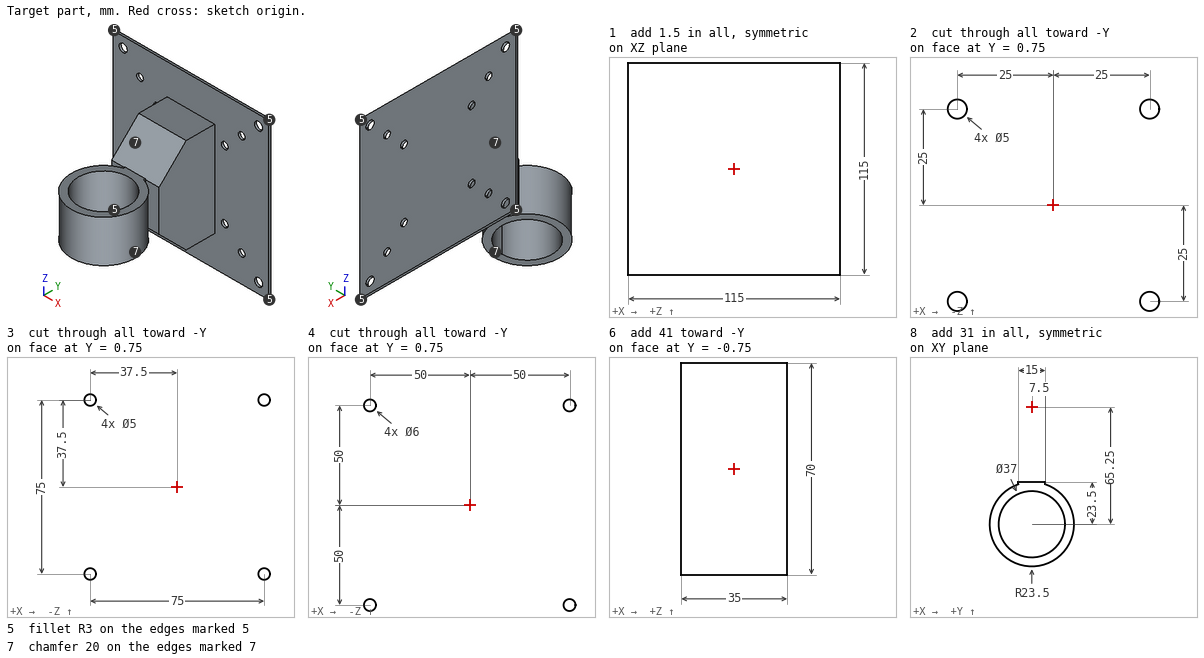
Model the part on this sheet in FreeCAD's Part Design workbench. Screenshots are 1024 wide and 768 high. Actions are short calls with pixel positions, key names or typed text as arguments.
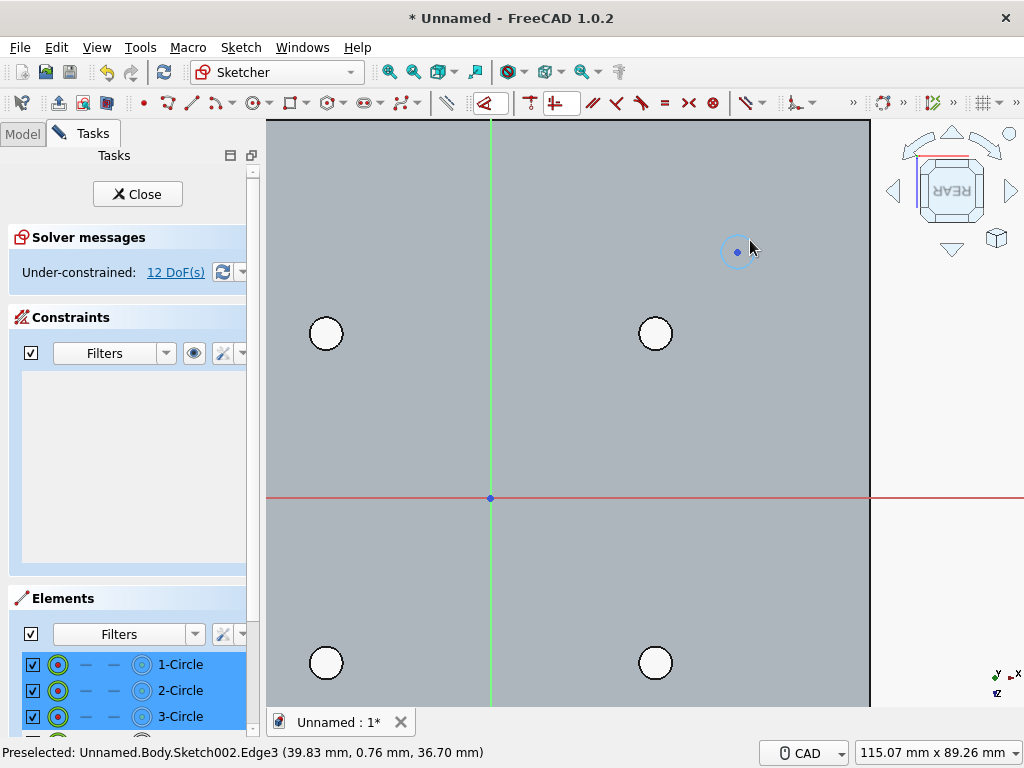
click(749, 240)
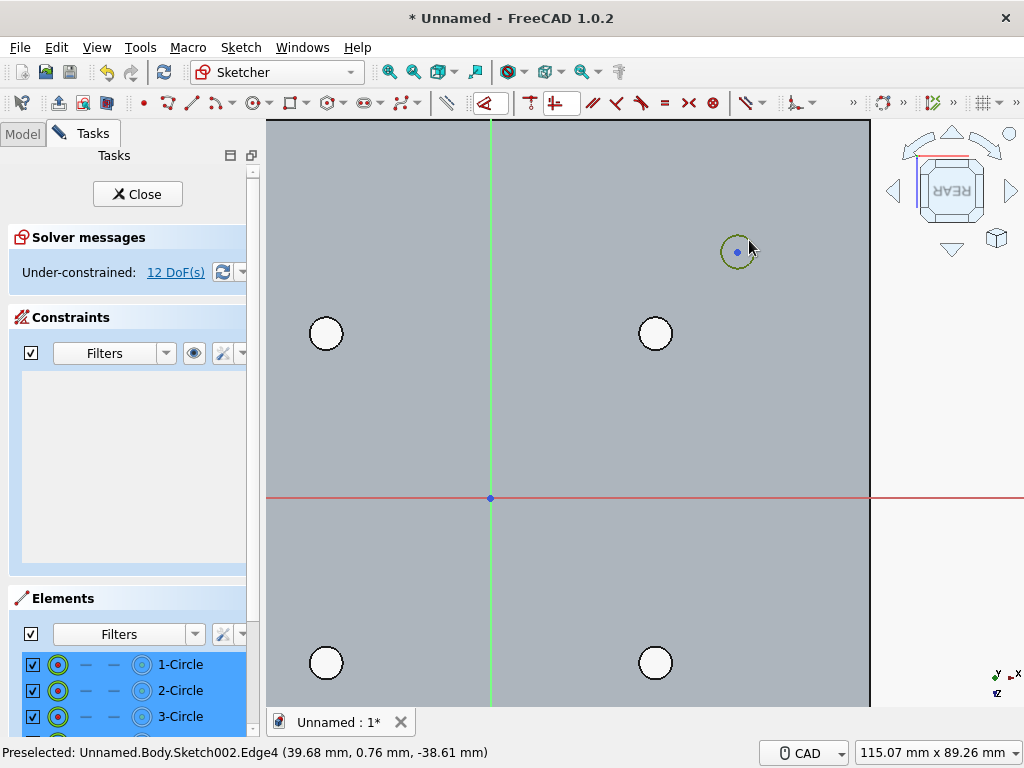
key(e)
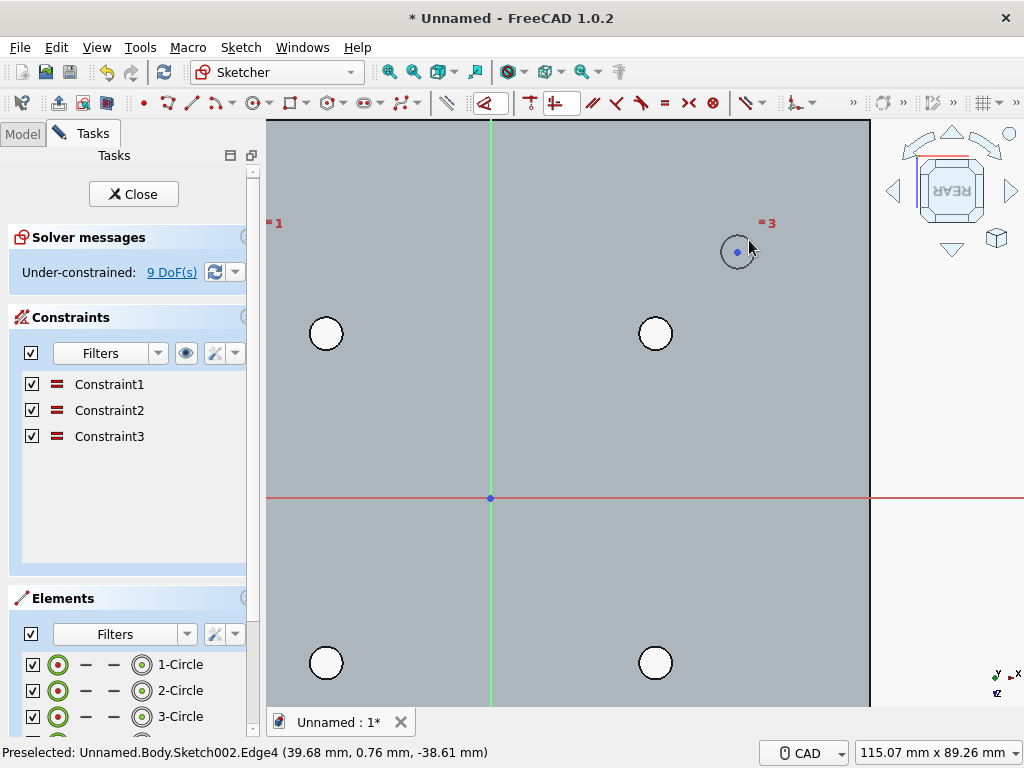
scroll(750, 239, down, 2)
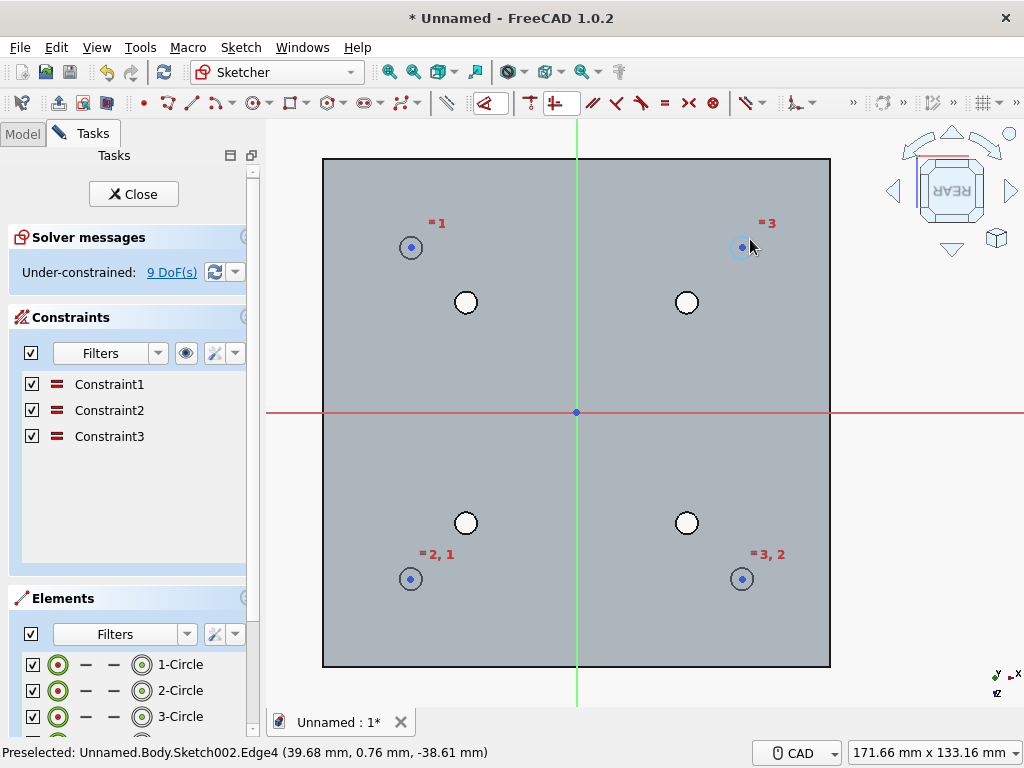
click(411, 248)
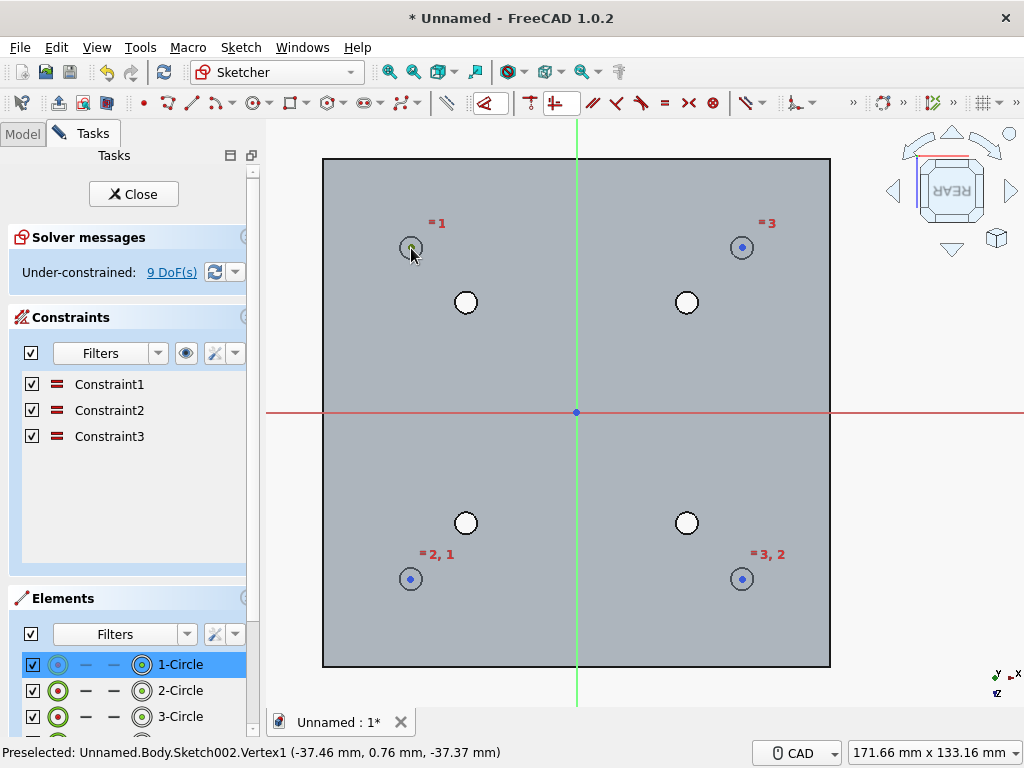
click(411, 579)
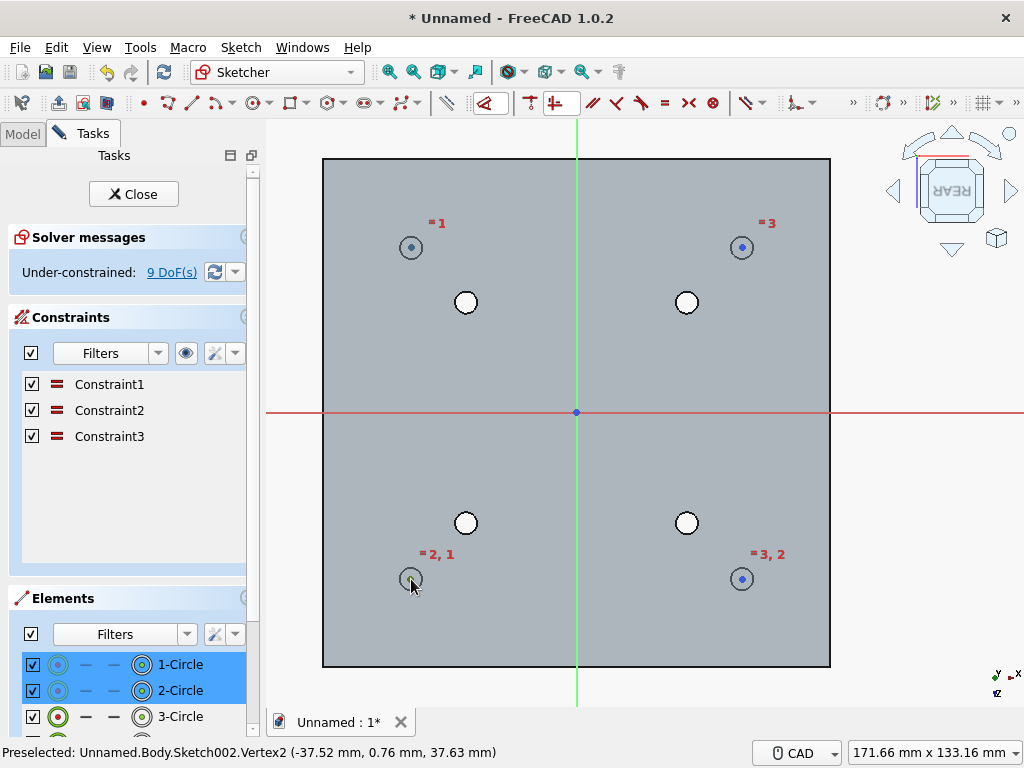
key(v)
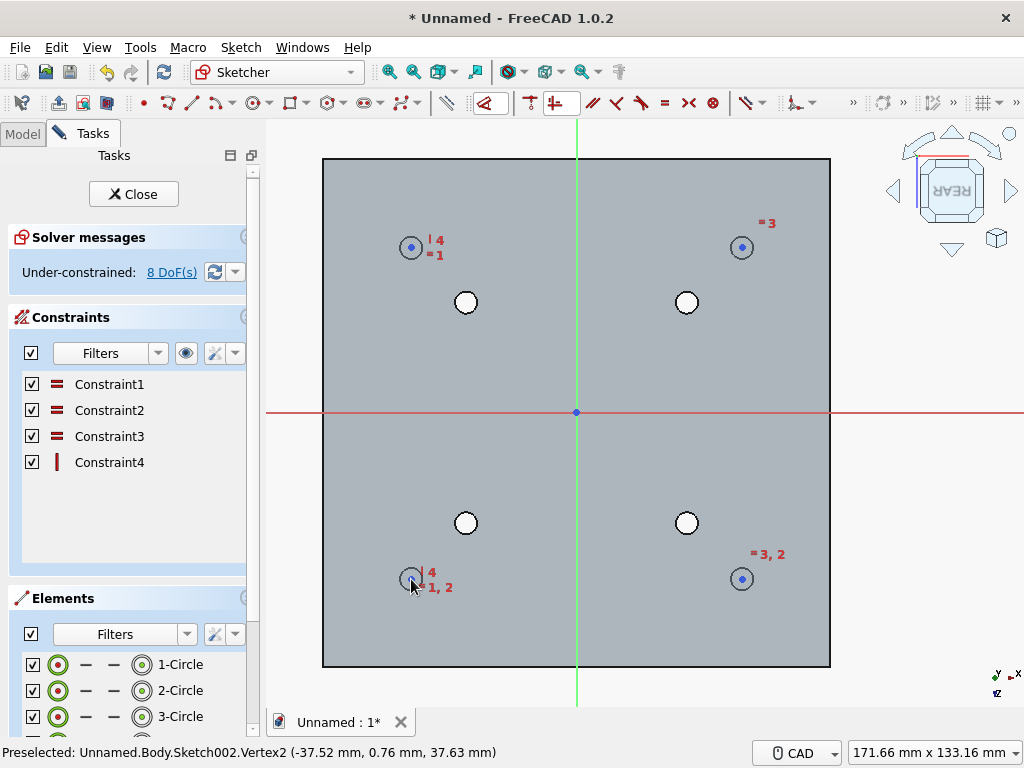
click(411, 579)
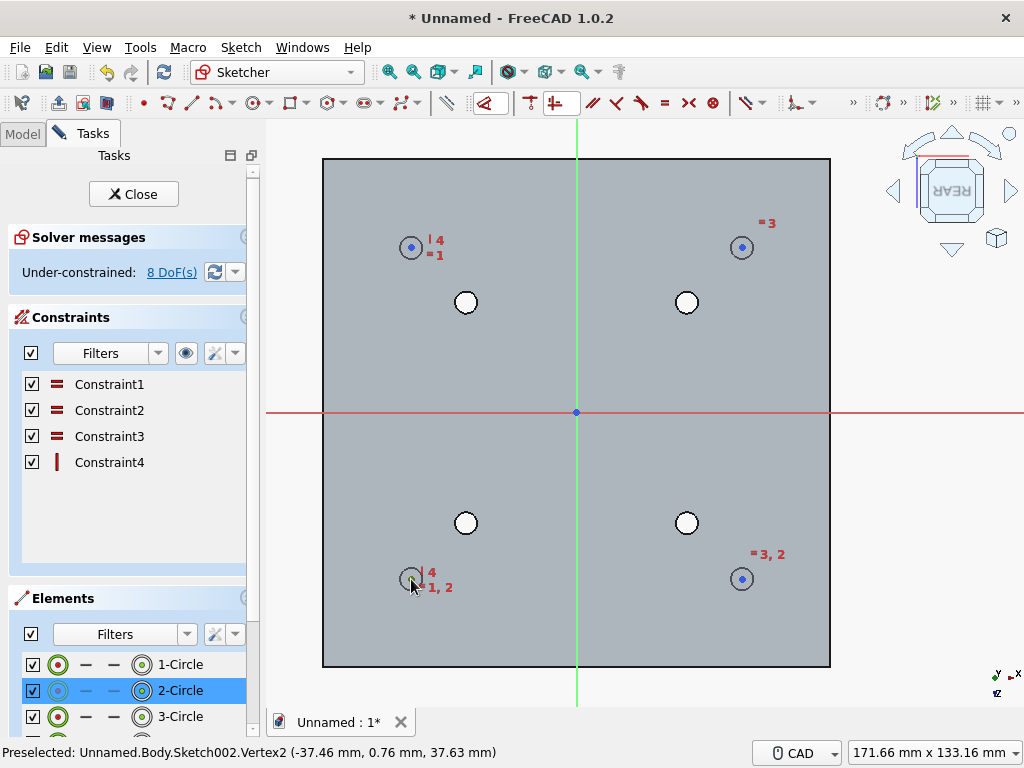
click(742, 579)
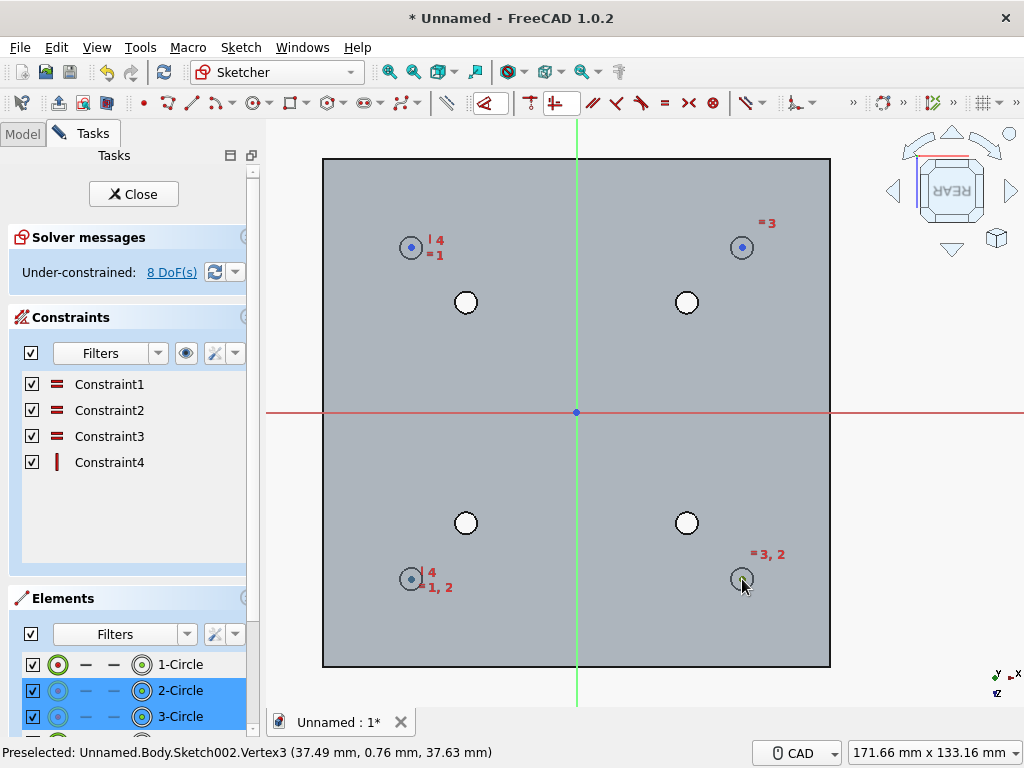
key(h)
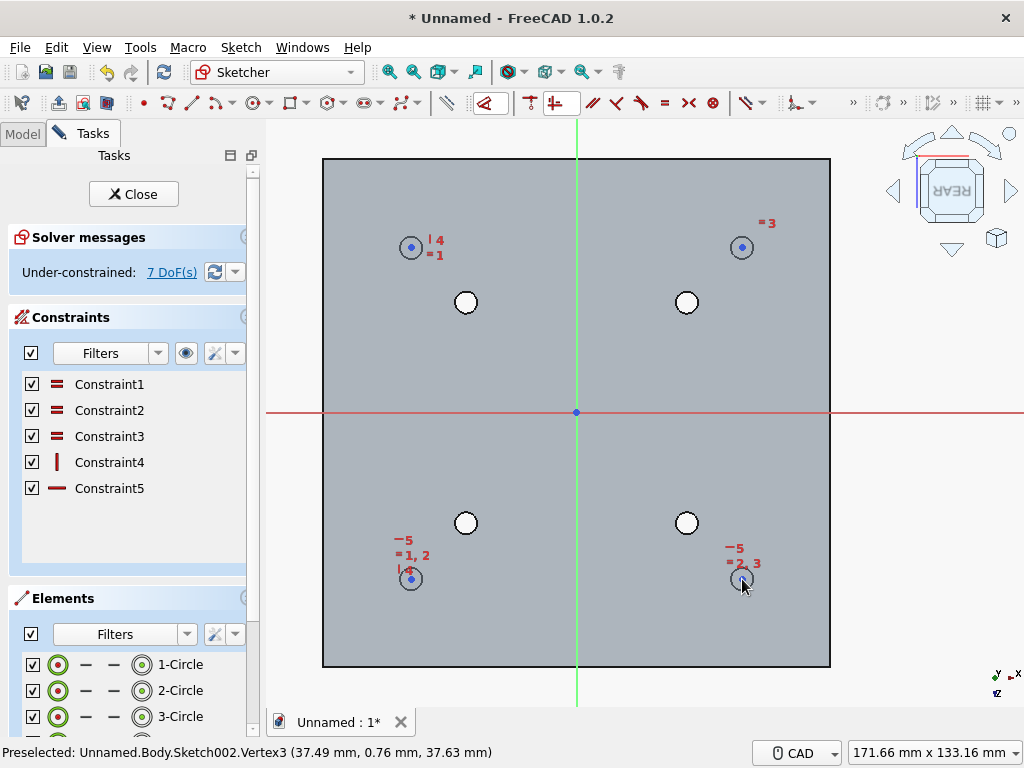
click(742, 579)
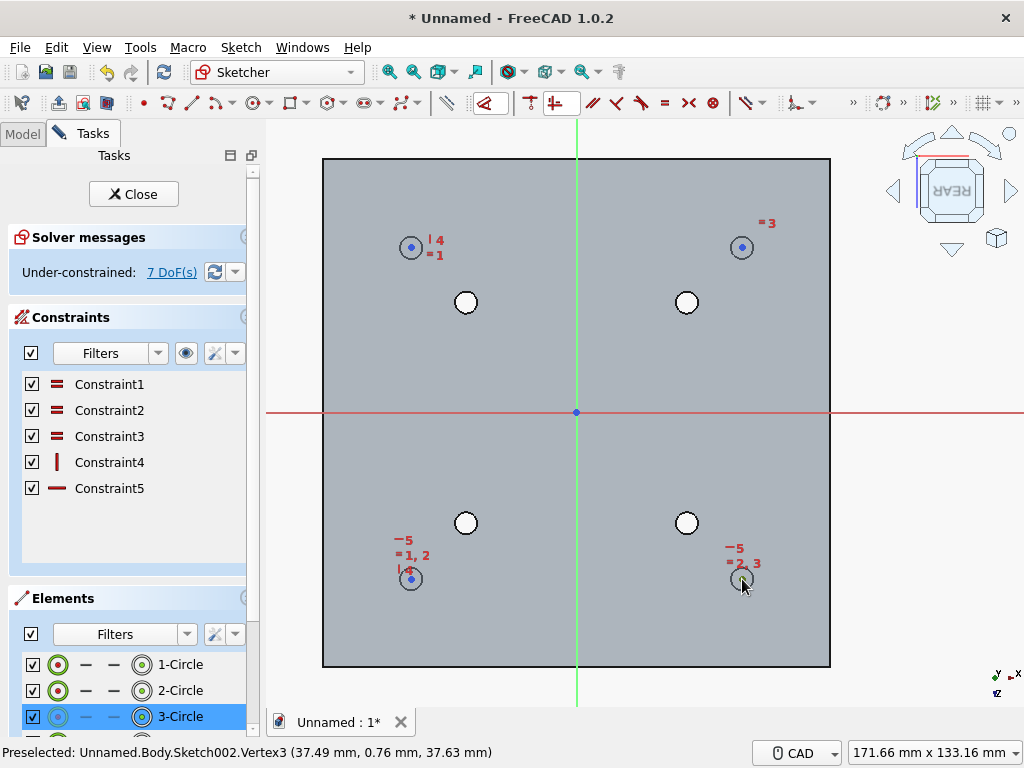
click(742, 248)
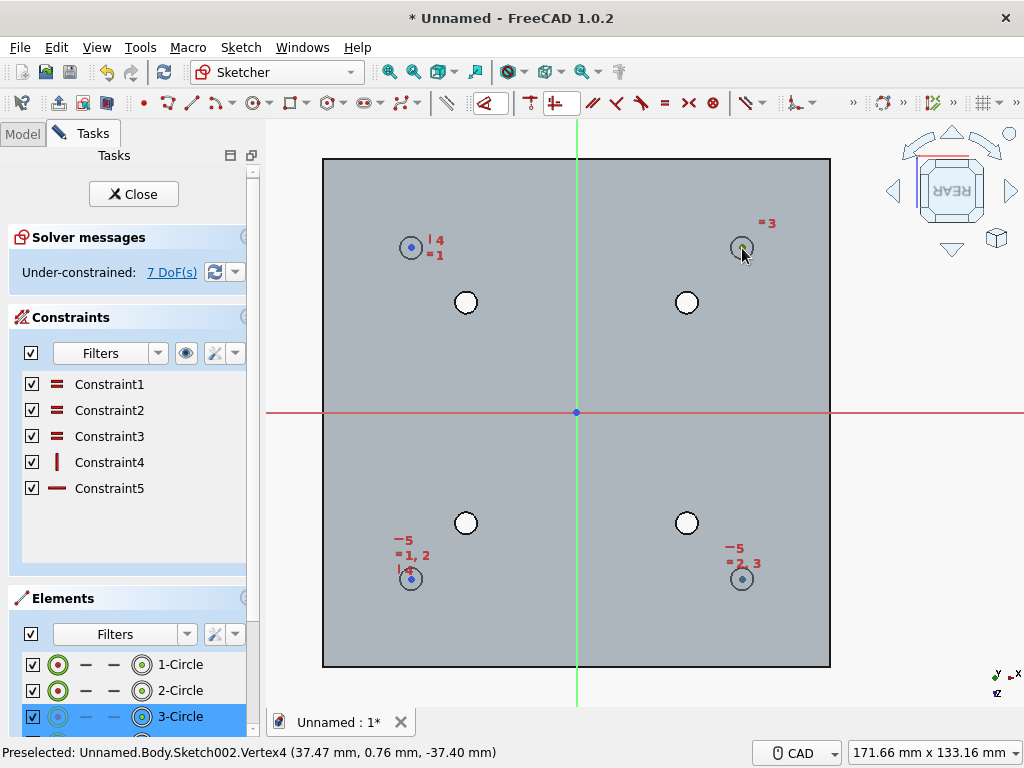
key(v)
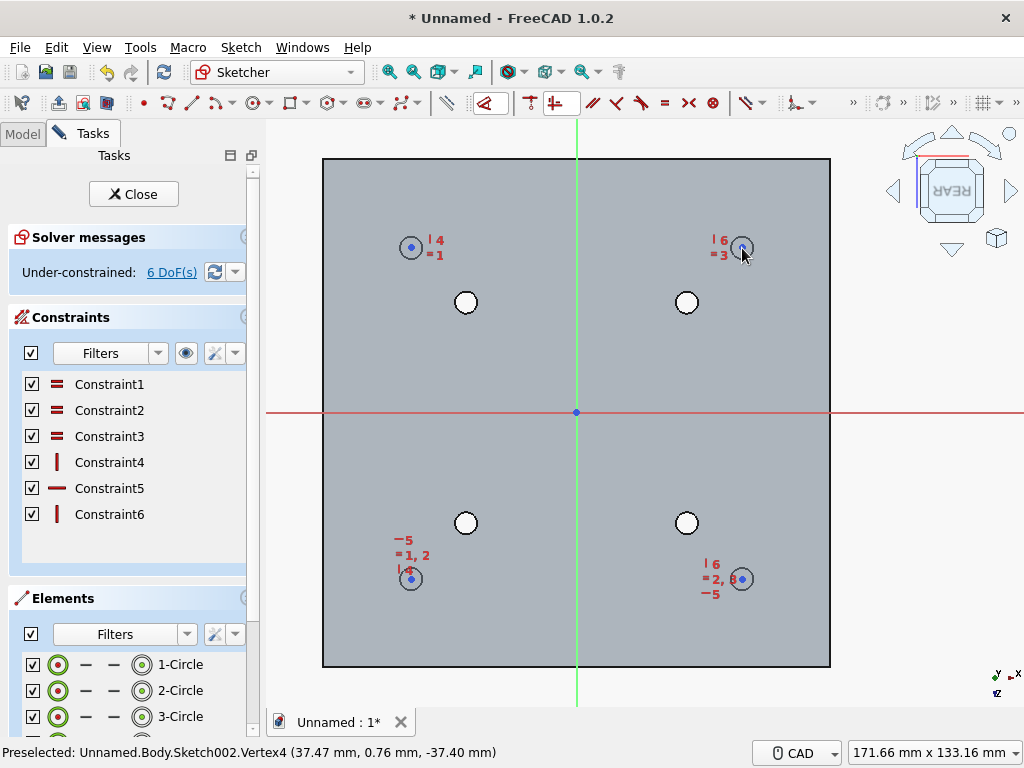
click(411, 248)